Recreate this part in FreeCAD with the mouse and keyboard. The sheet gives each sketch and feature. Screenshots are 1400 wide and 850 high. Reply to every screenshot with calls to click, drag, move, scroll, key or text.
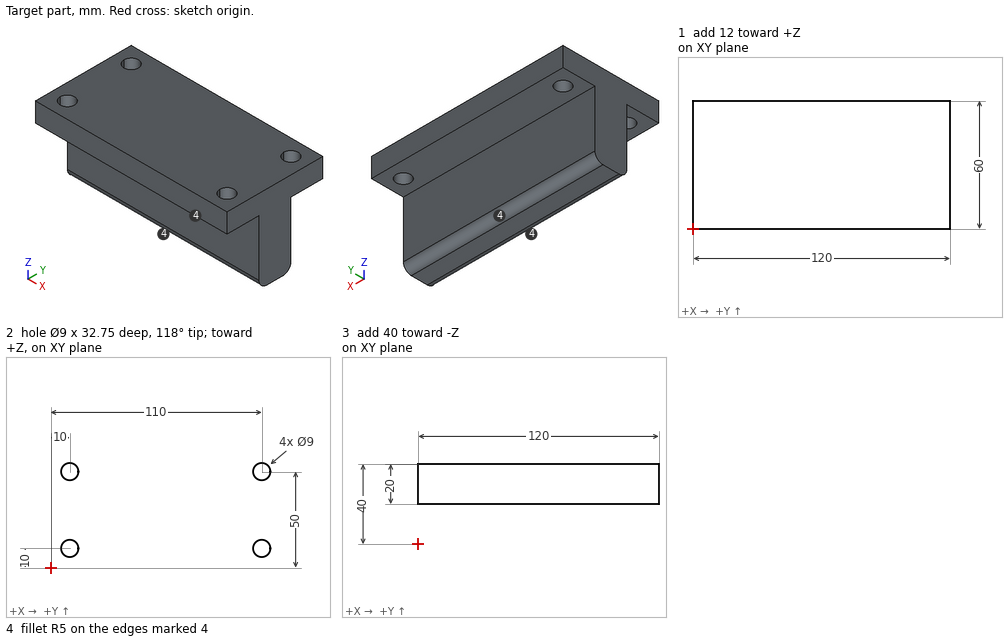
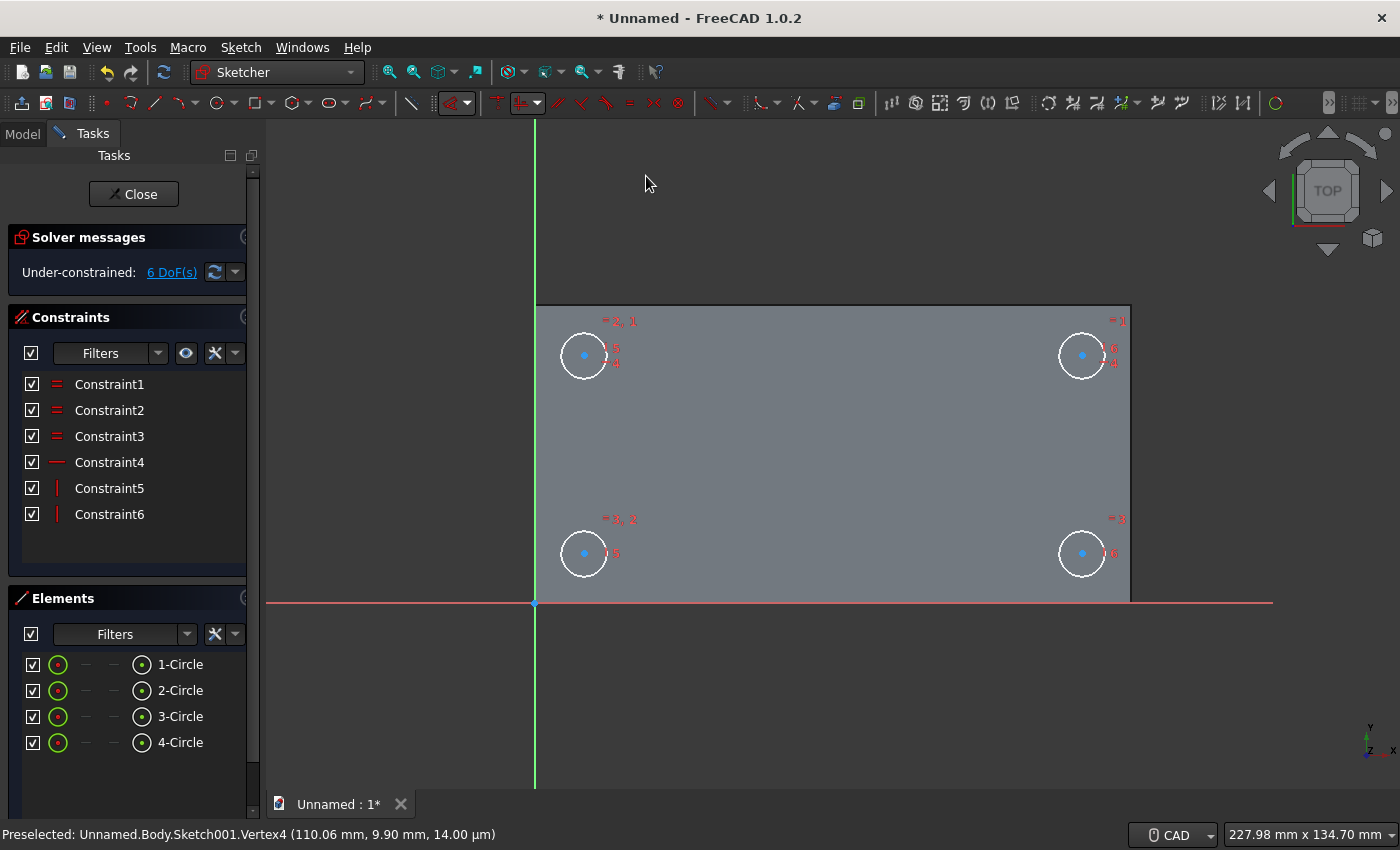
click(584, 554)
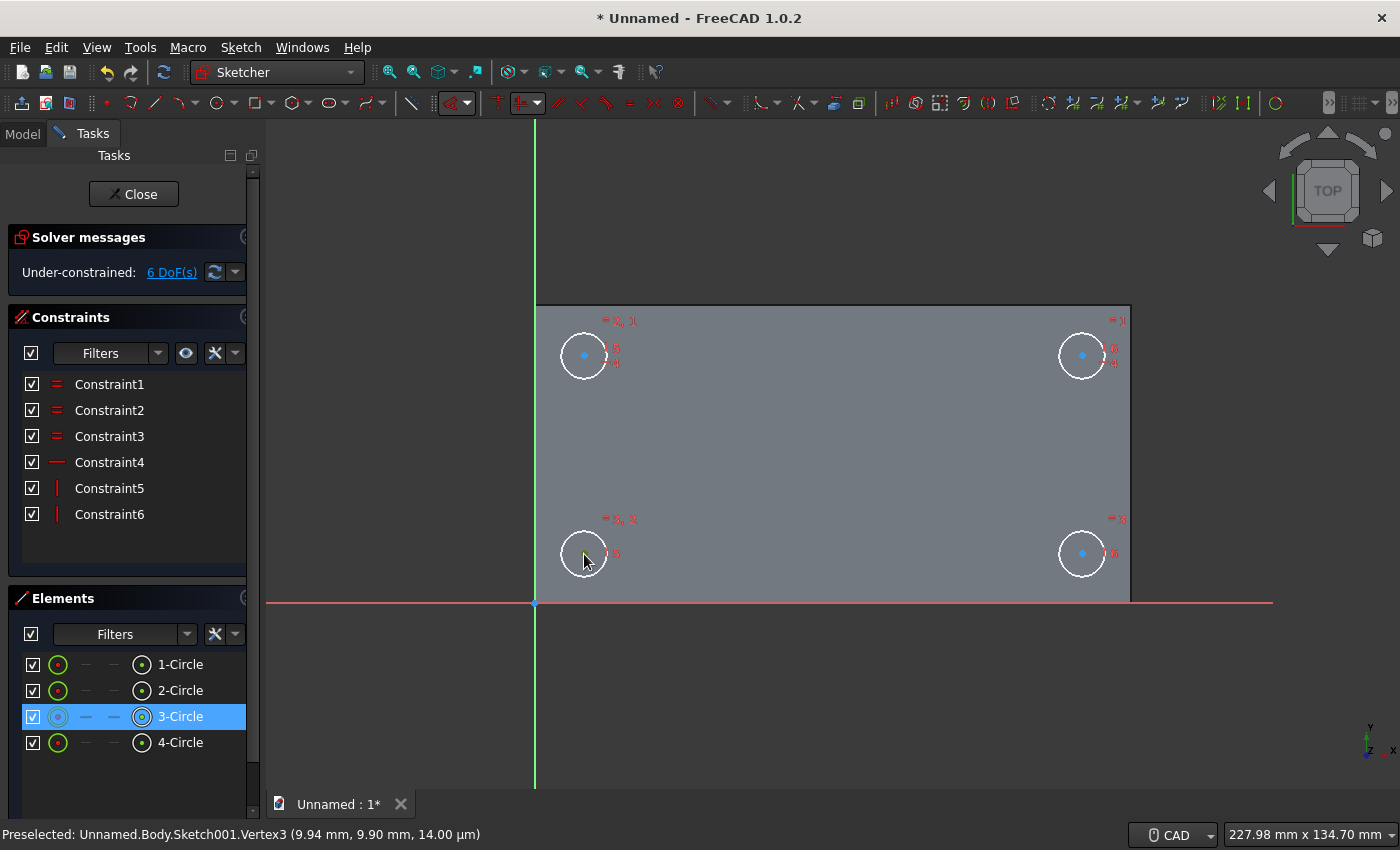
click(1082, 554)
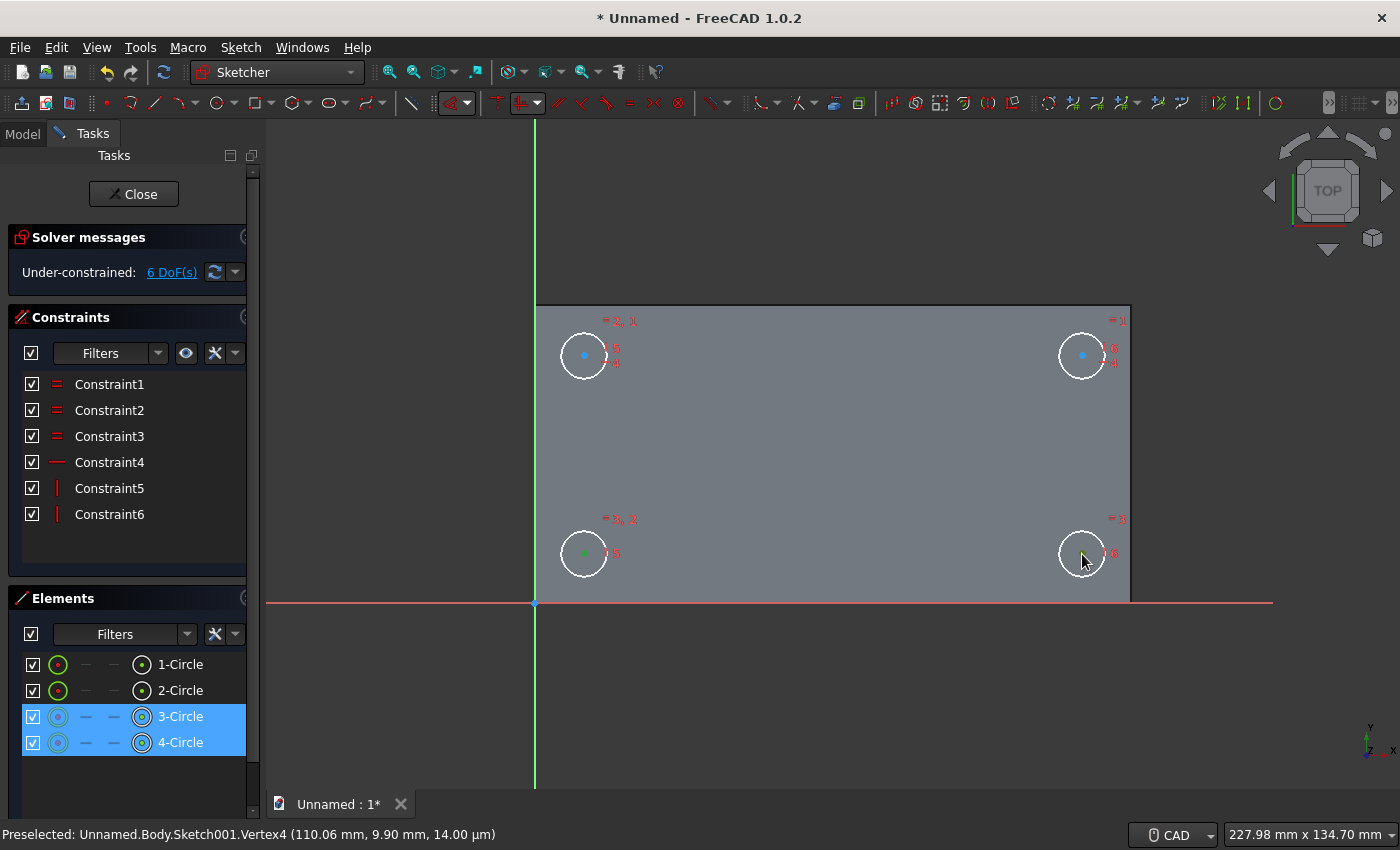
key(h)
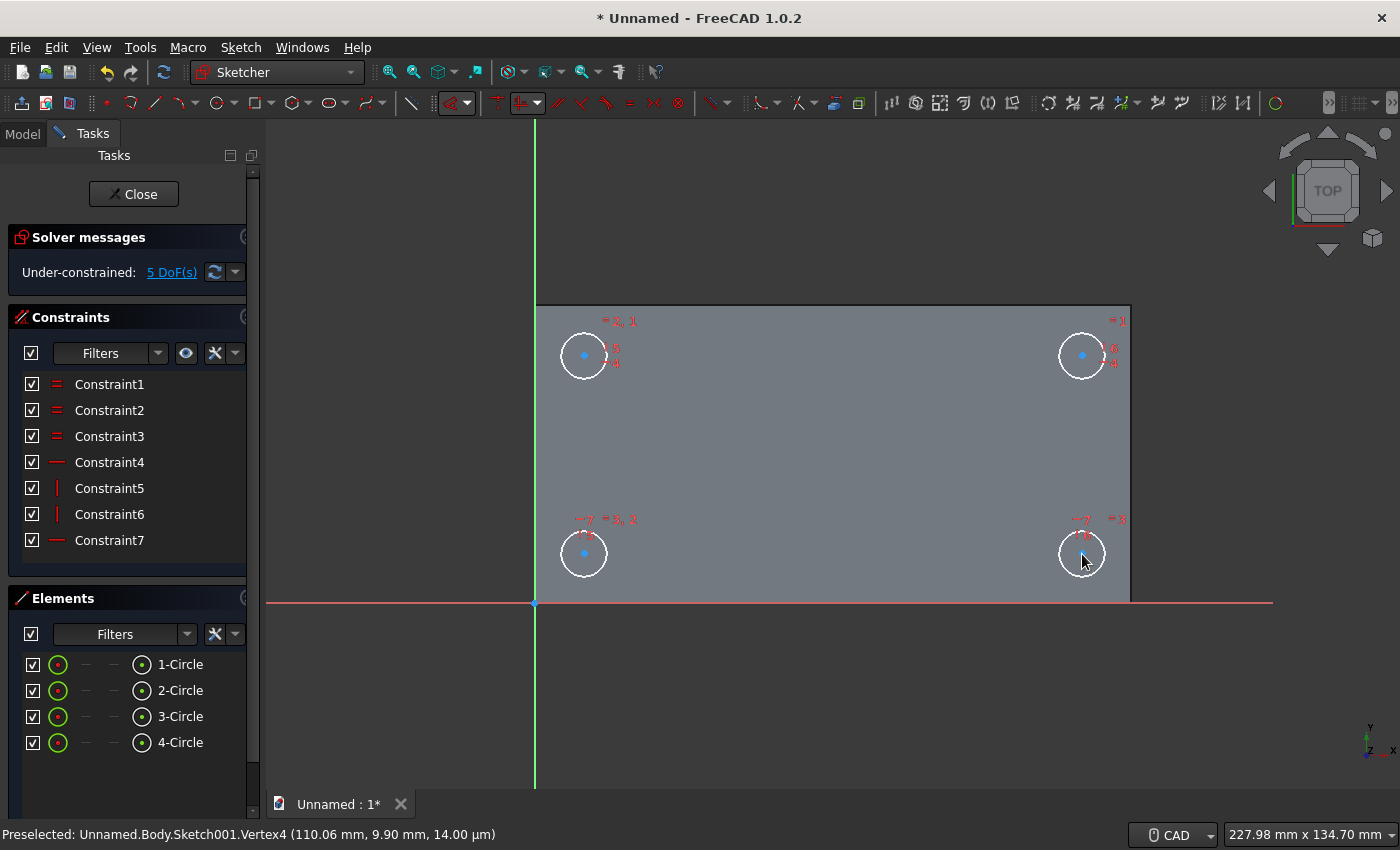
click(1098, 340)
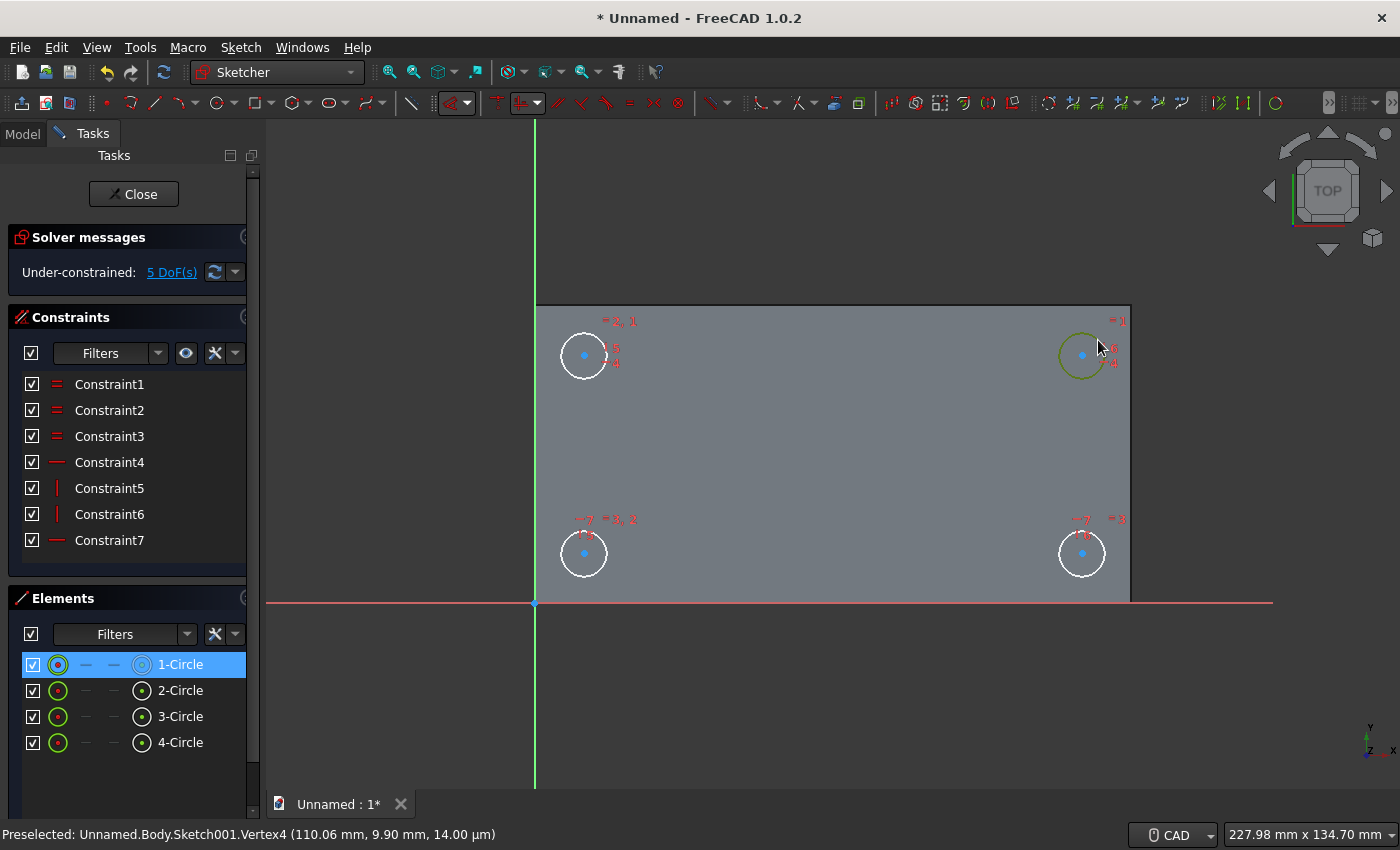
click(470, 104)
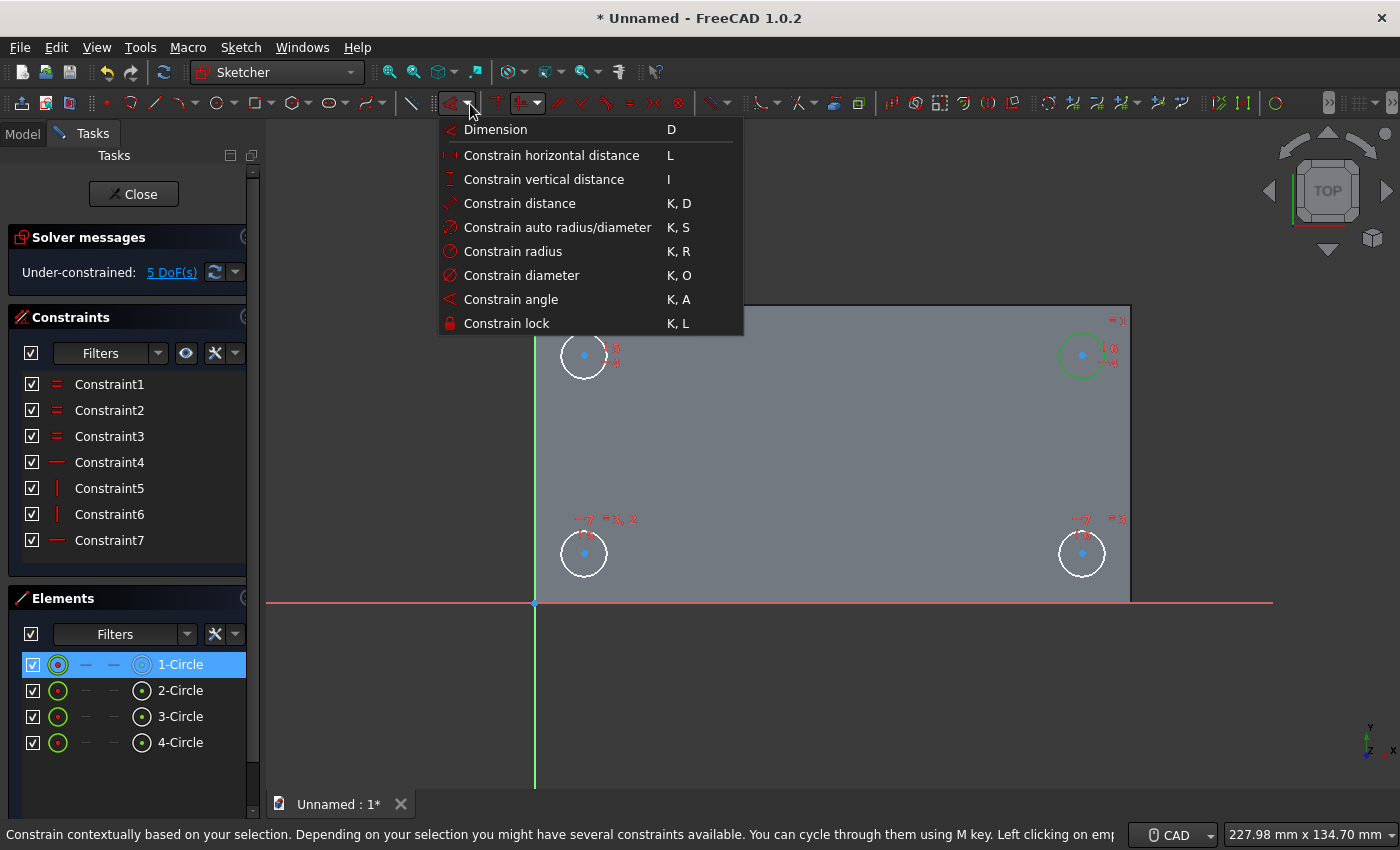
click(591, 275)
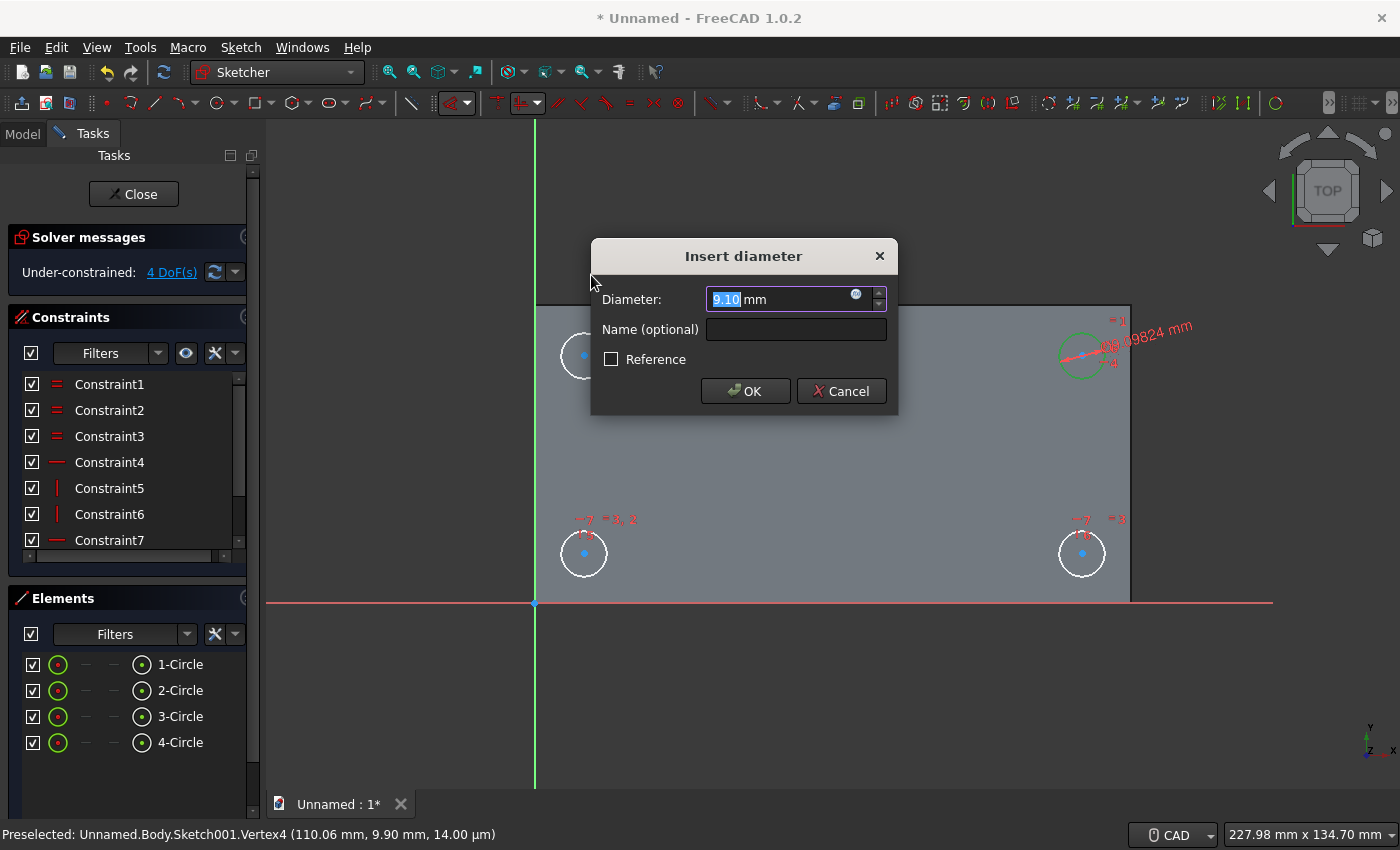
text(9)
key(Return)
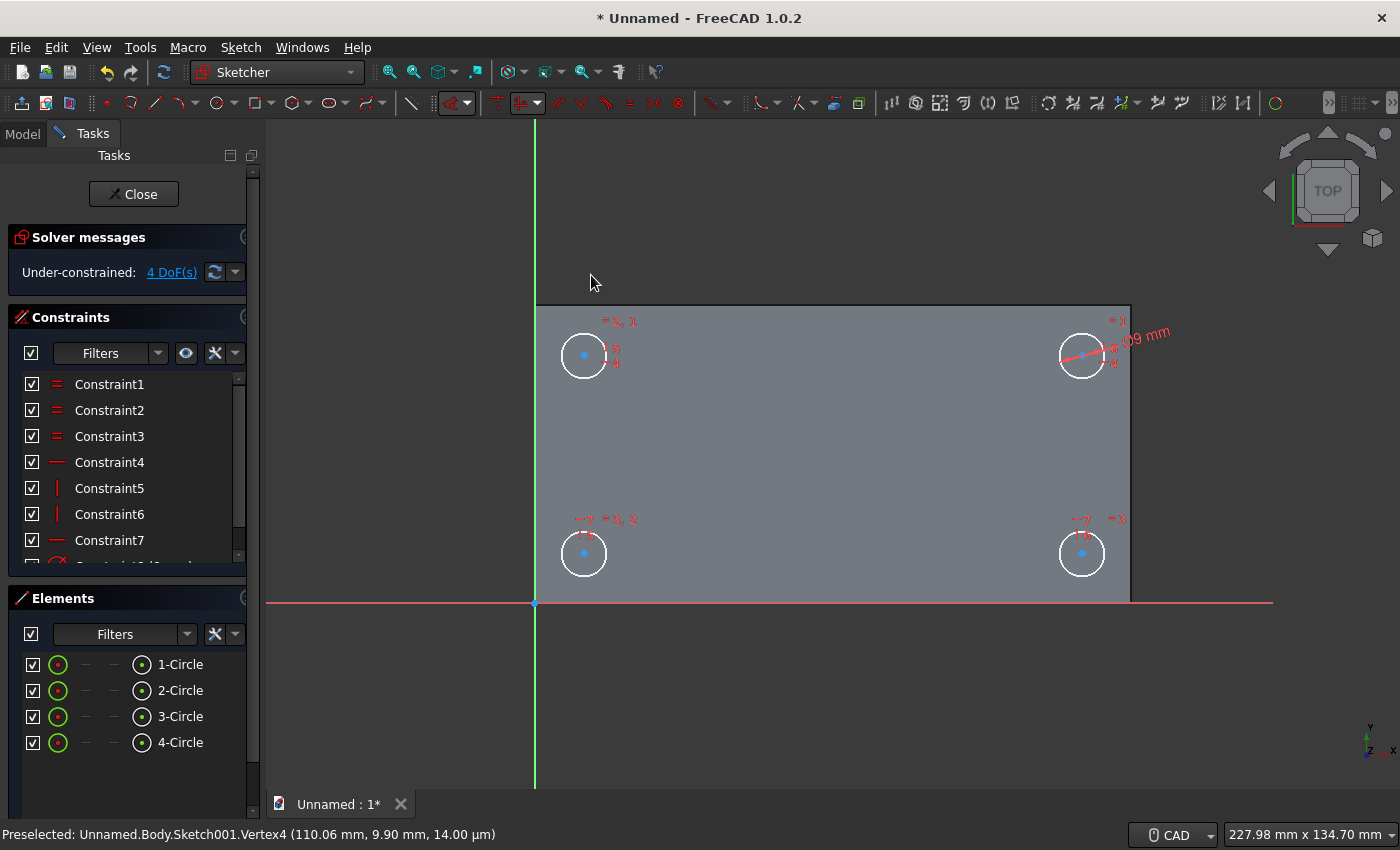
click(1082, 356)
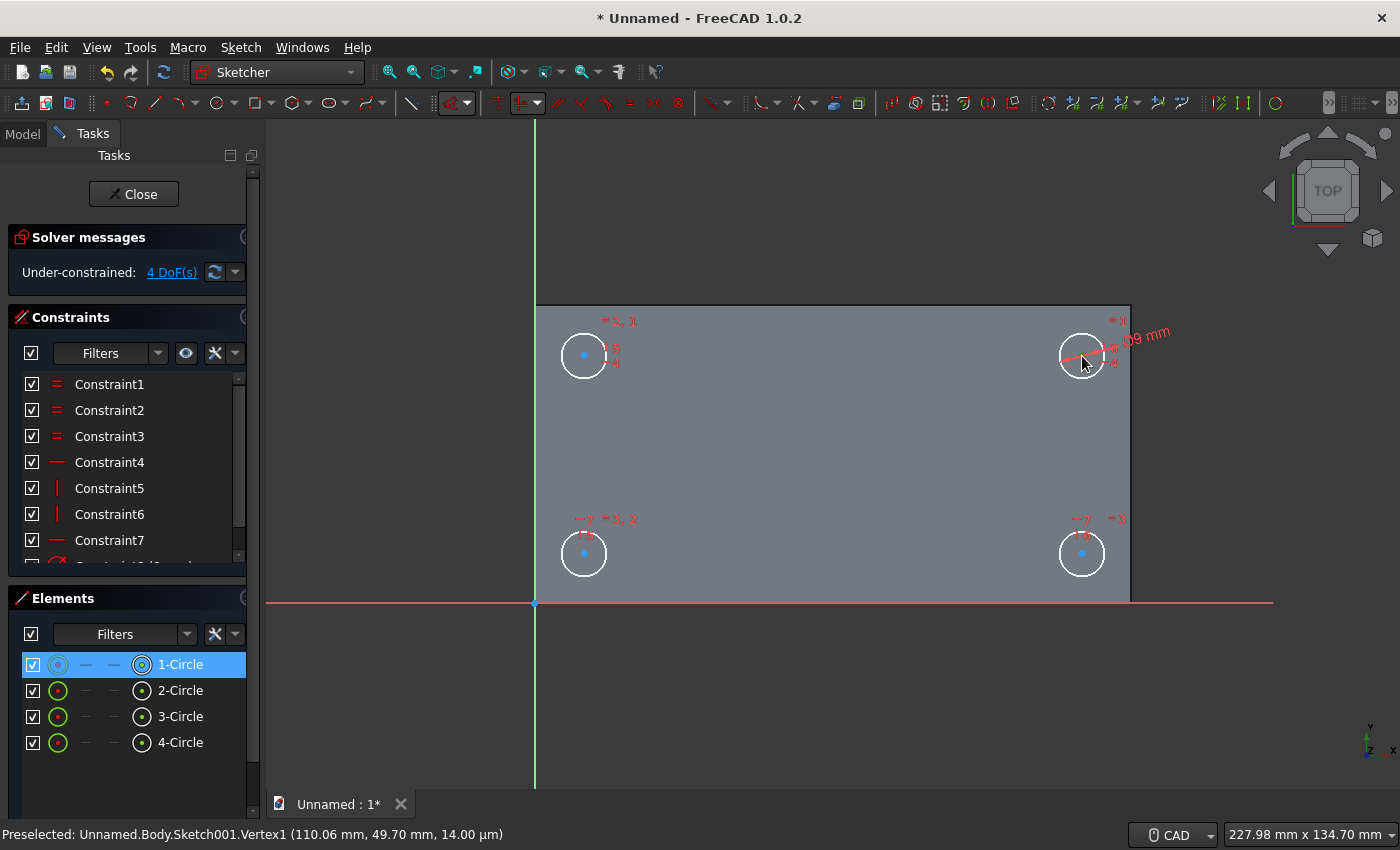
click(470, 104)